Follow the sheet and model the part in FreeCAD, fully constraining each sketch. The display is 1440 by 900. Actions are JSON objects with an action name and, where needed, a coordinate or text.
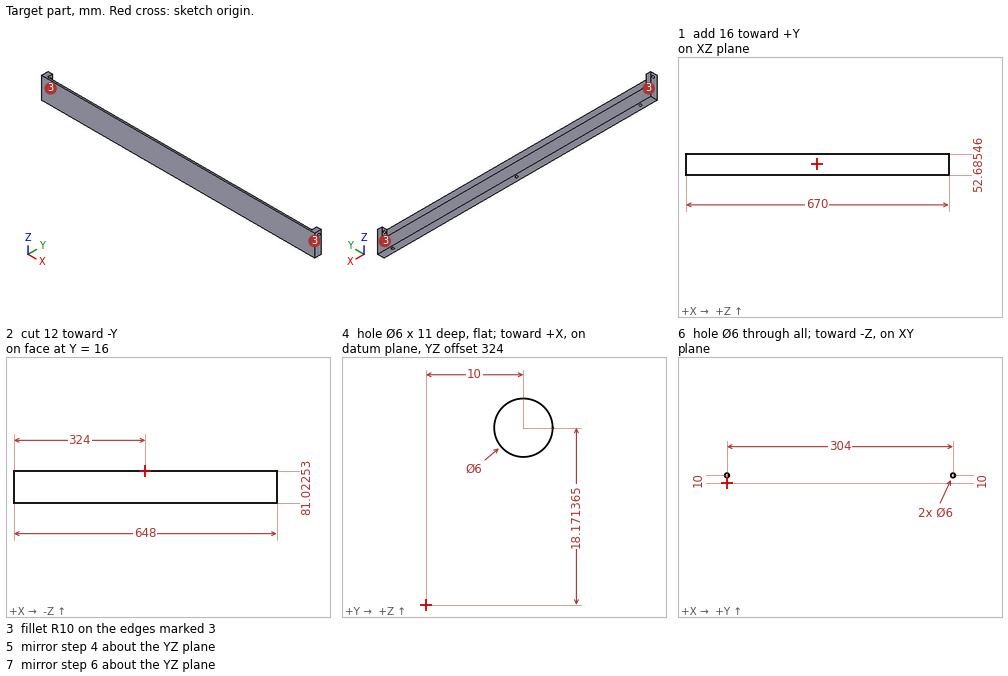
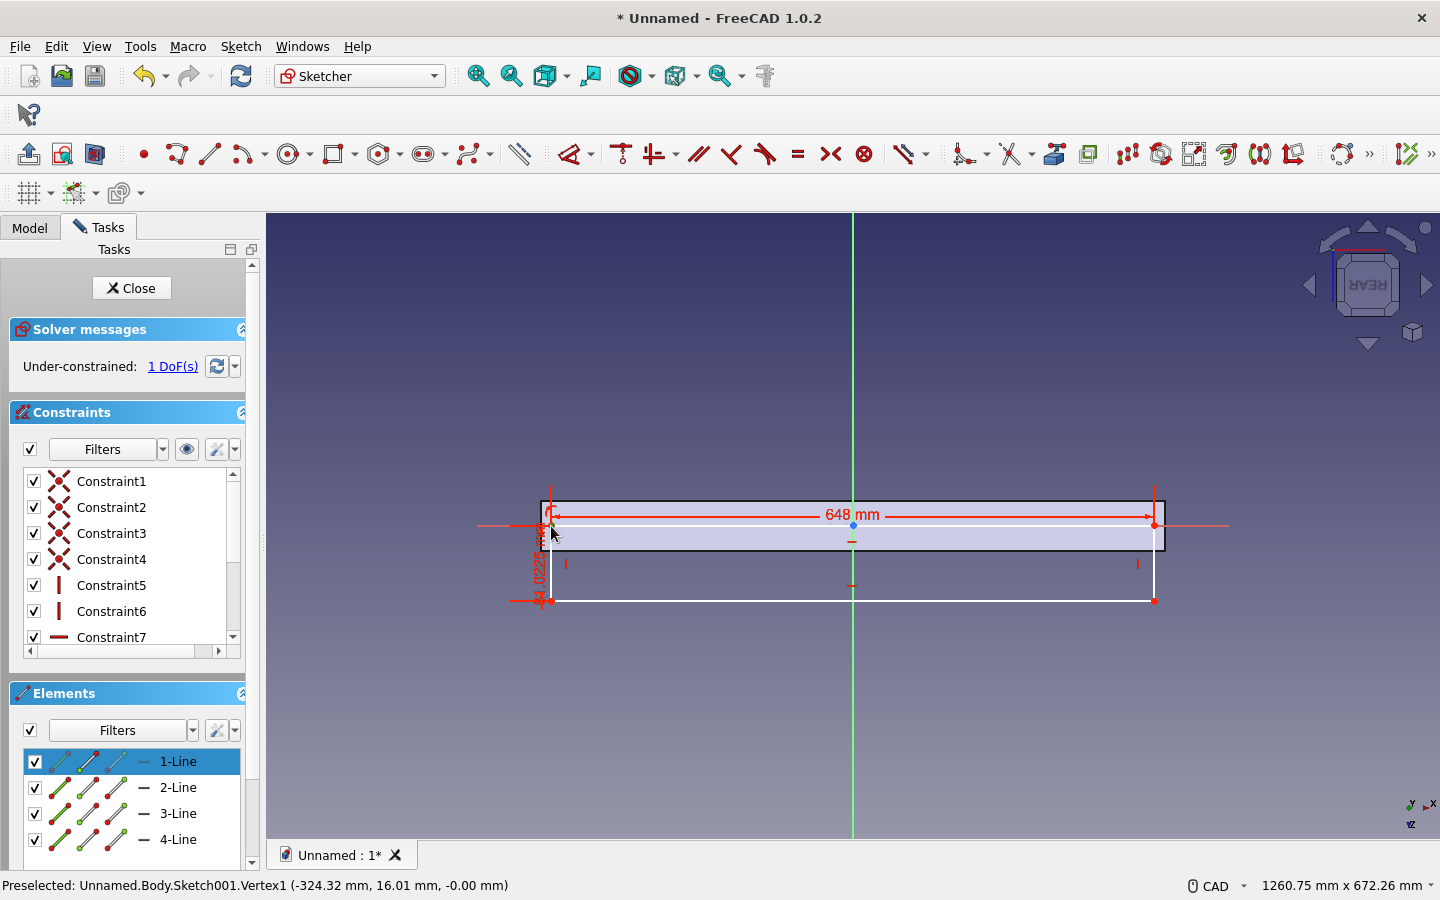
{"action": "key", "text": "l"}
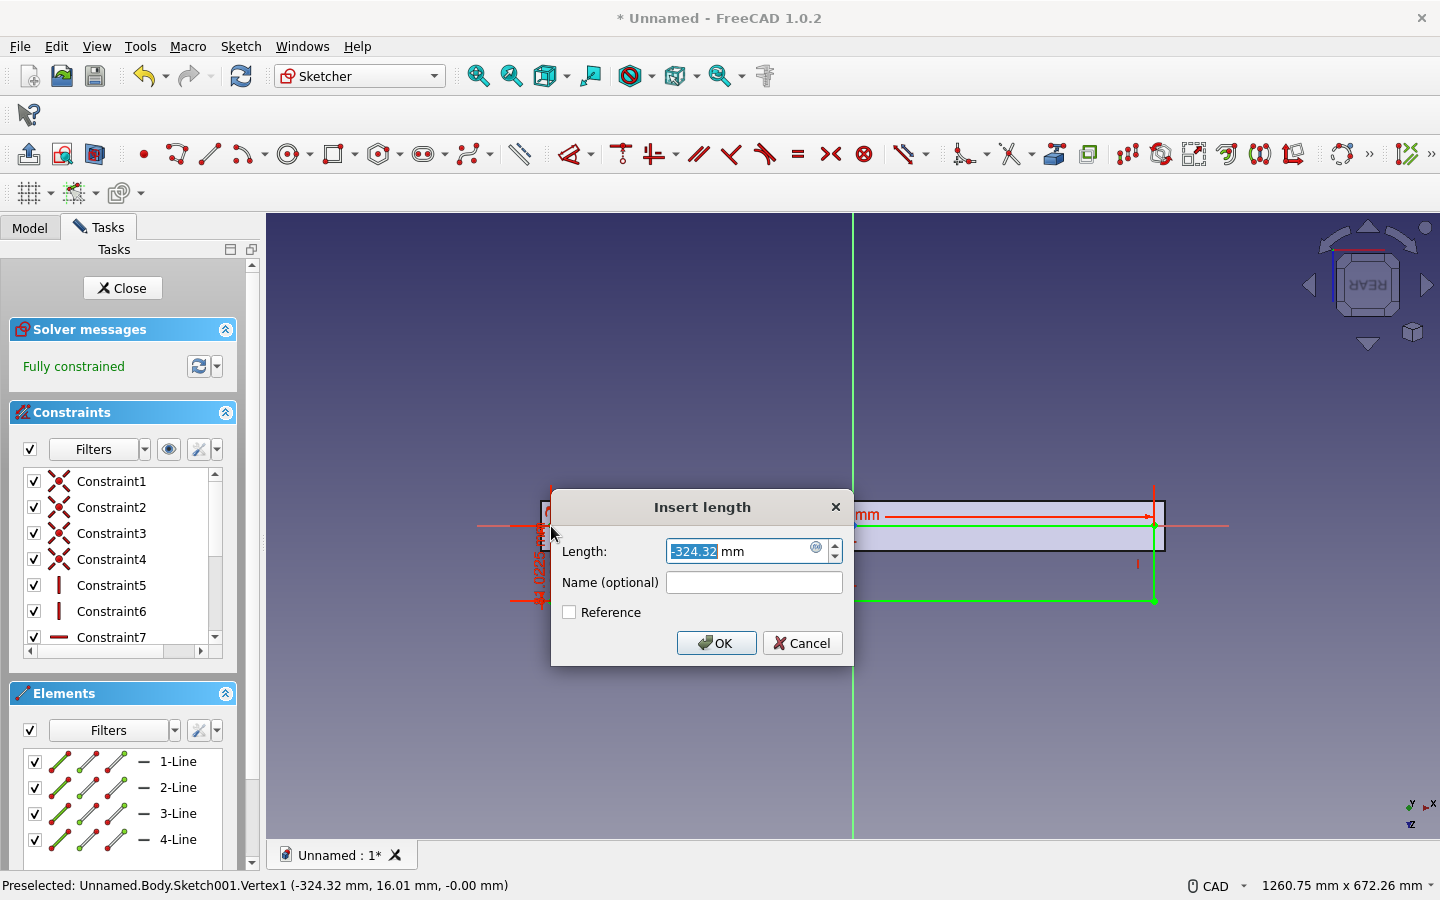
{"action": "type", "text": "-324"}
{"action": "key", "text": "Return"}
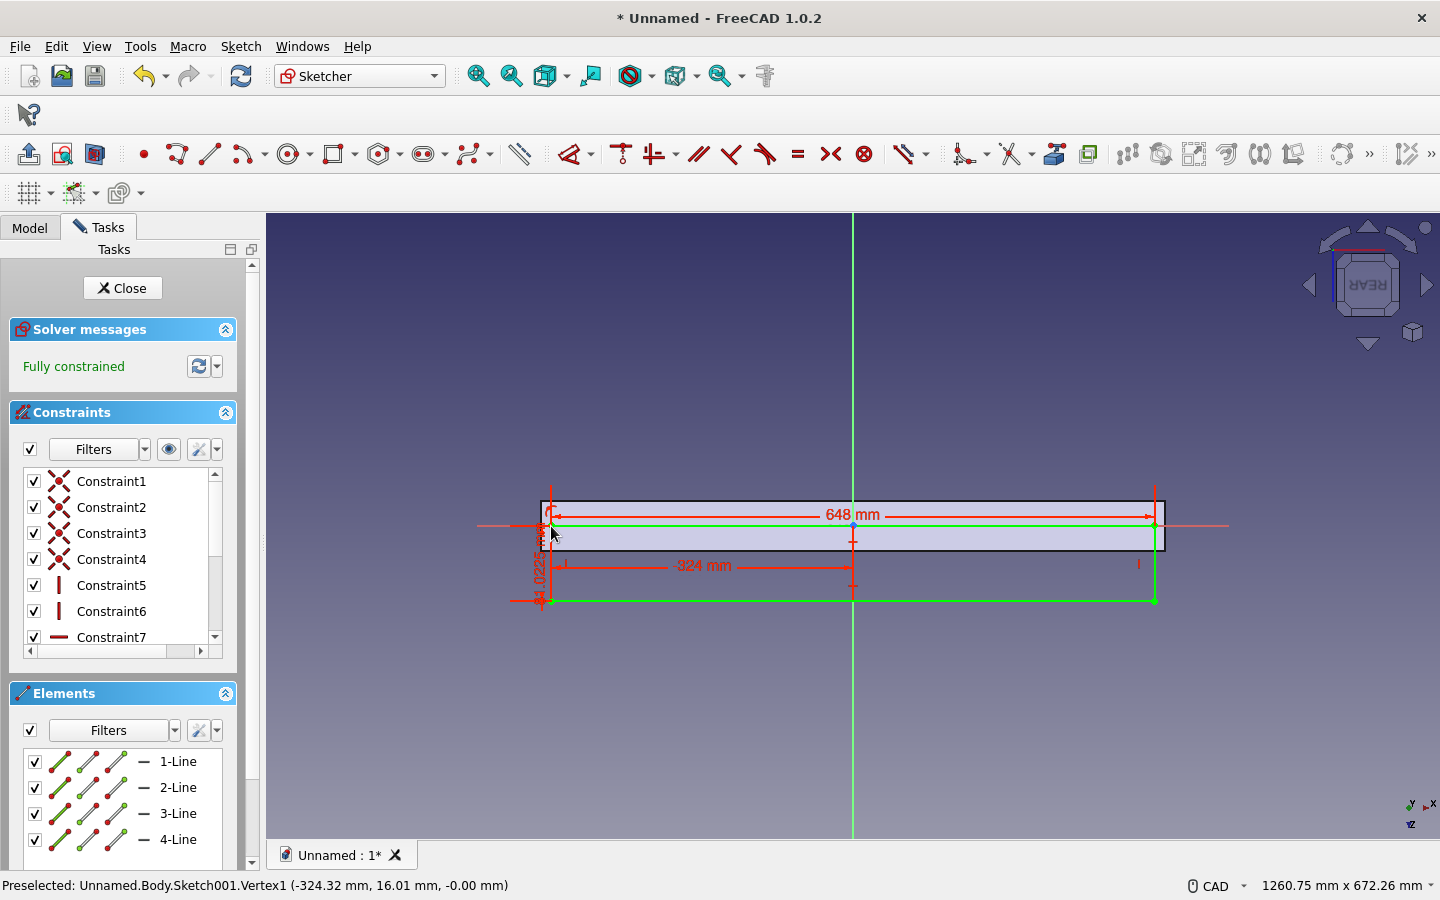
{"action": "left_click", "coordinate": [123, 288]}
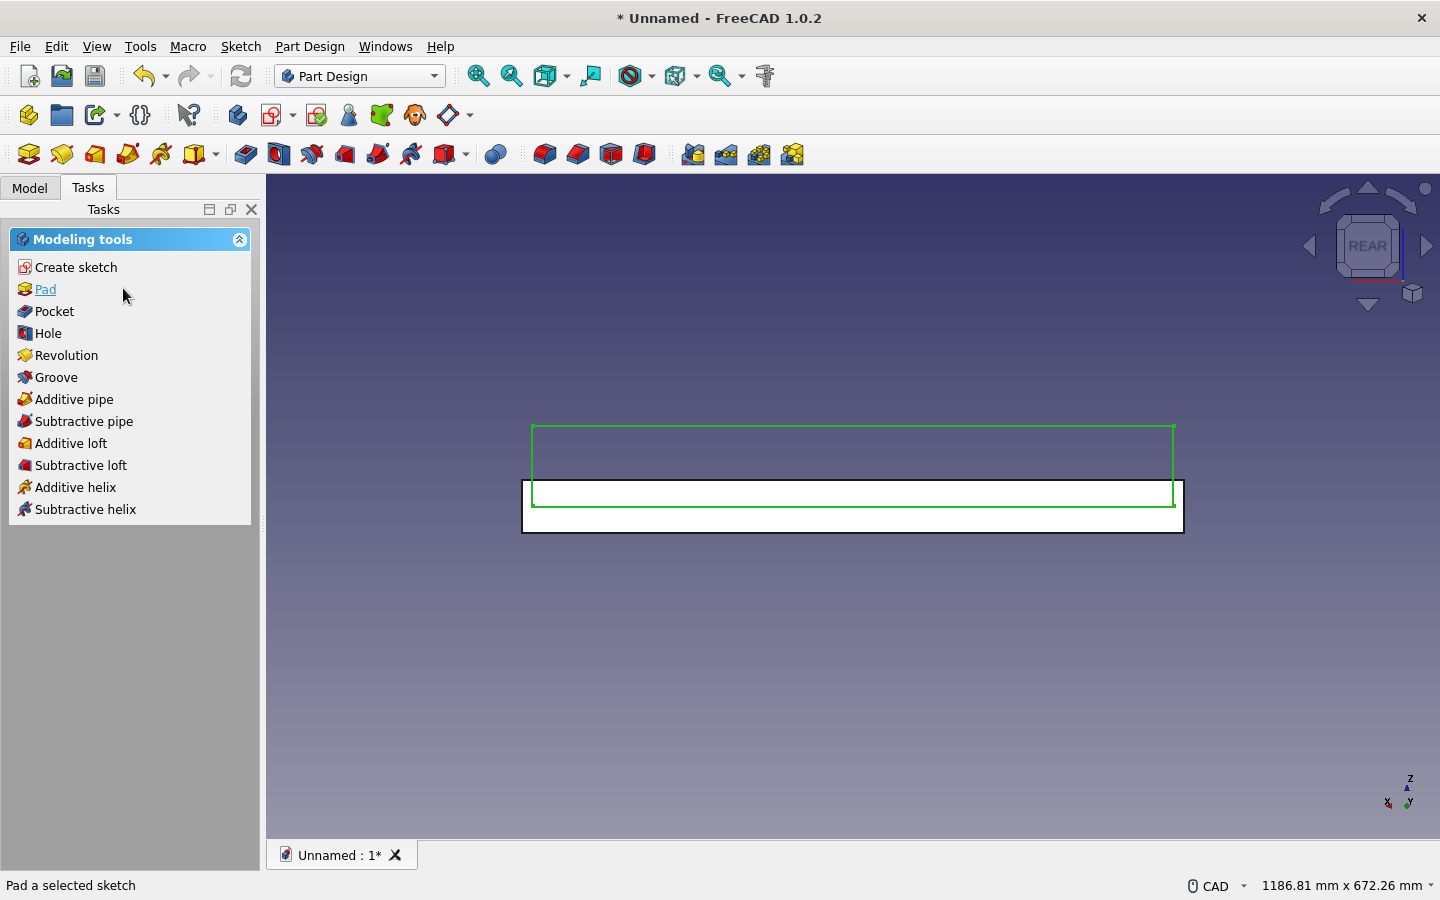
{"action": "left_click", "coordinate": [246, 154]}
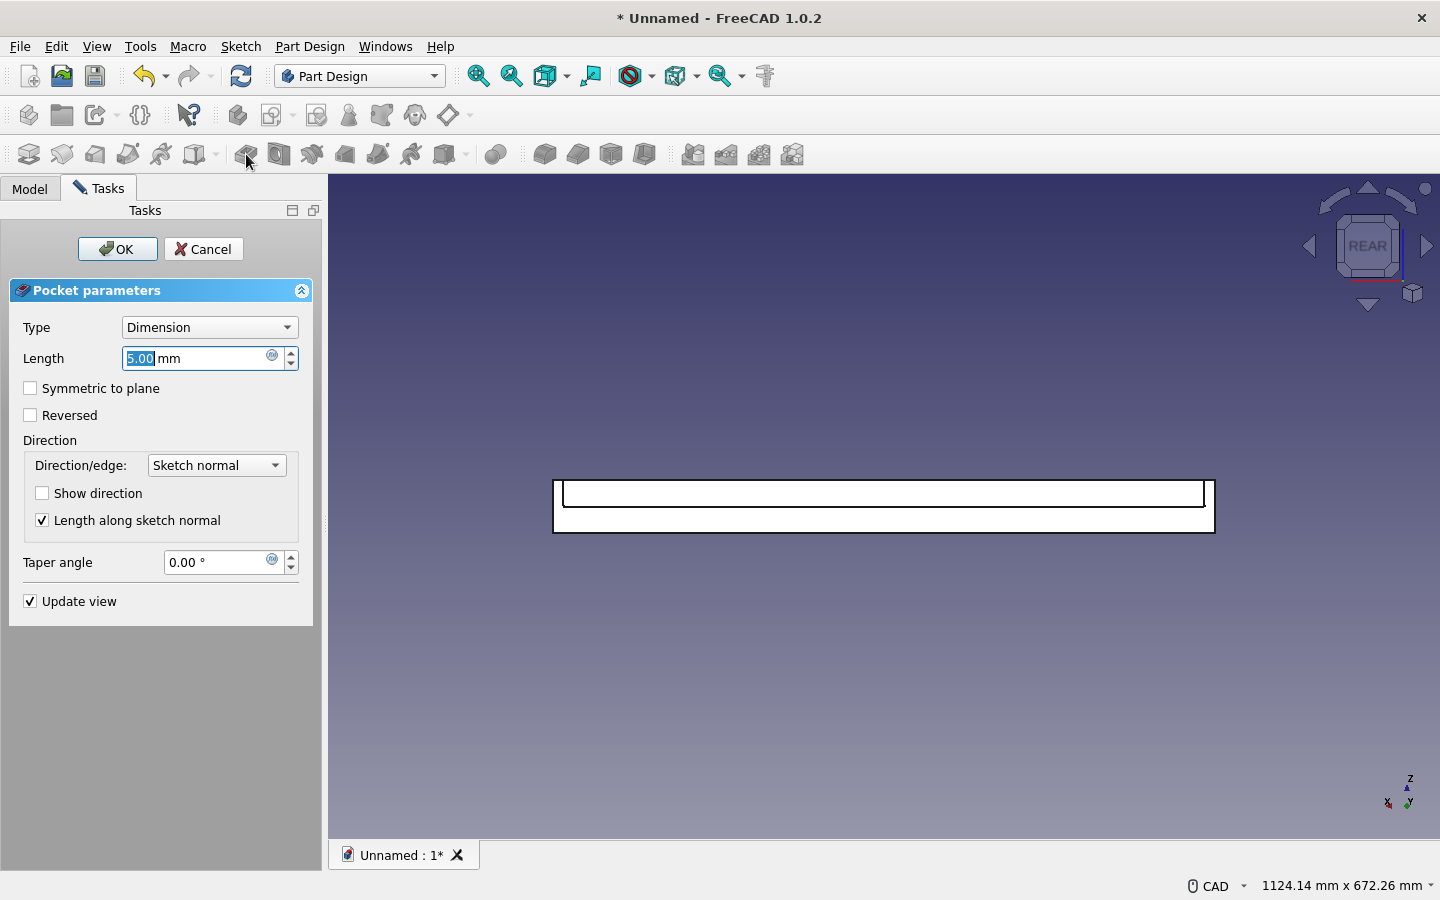
{"action": "type", "text": "12"}
{"action": "key", "text": "Tab"}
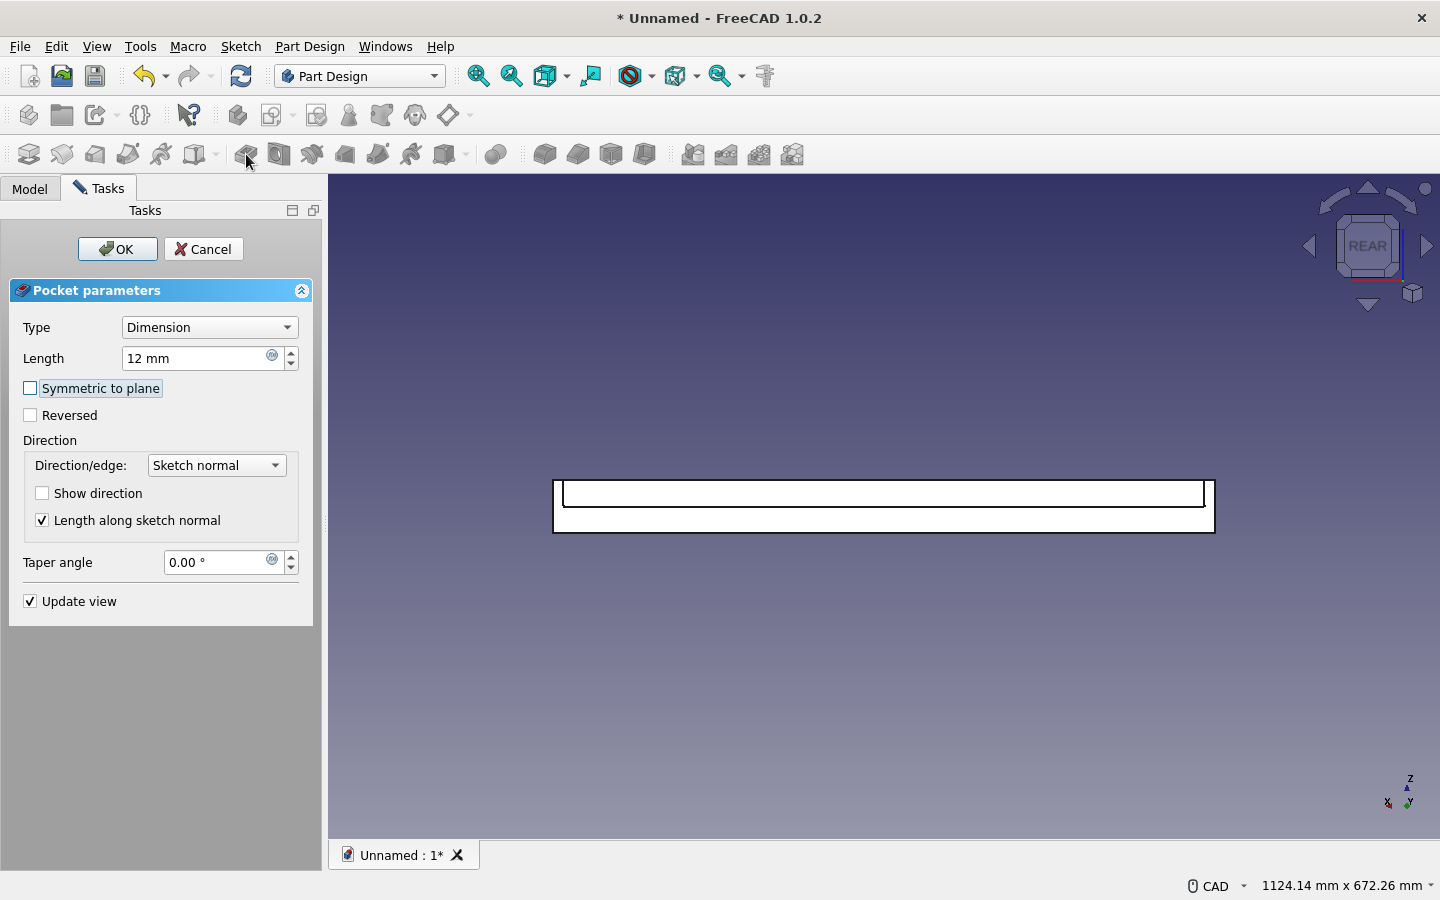
{"action": "left_click", "coordinate": [118, 249]}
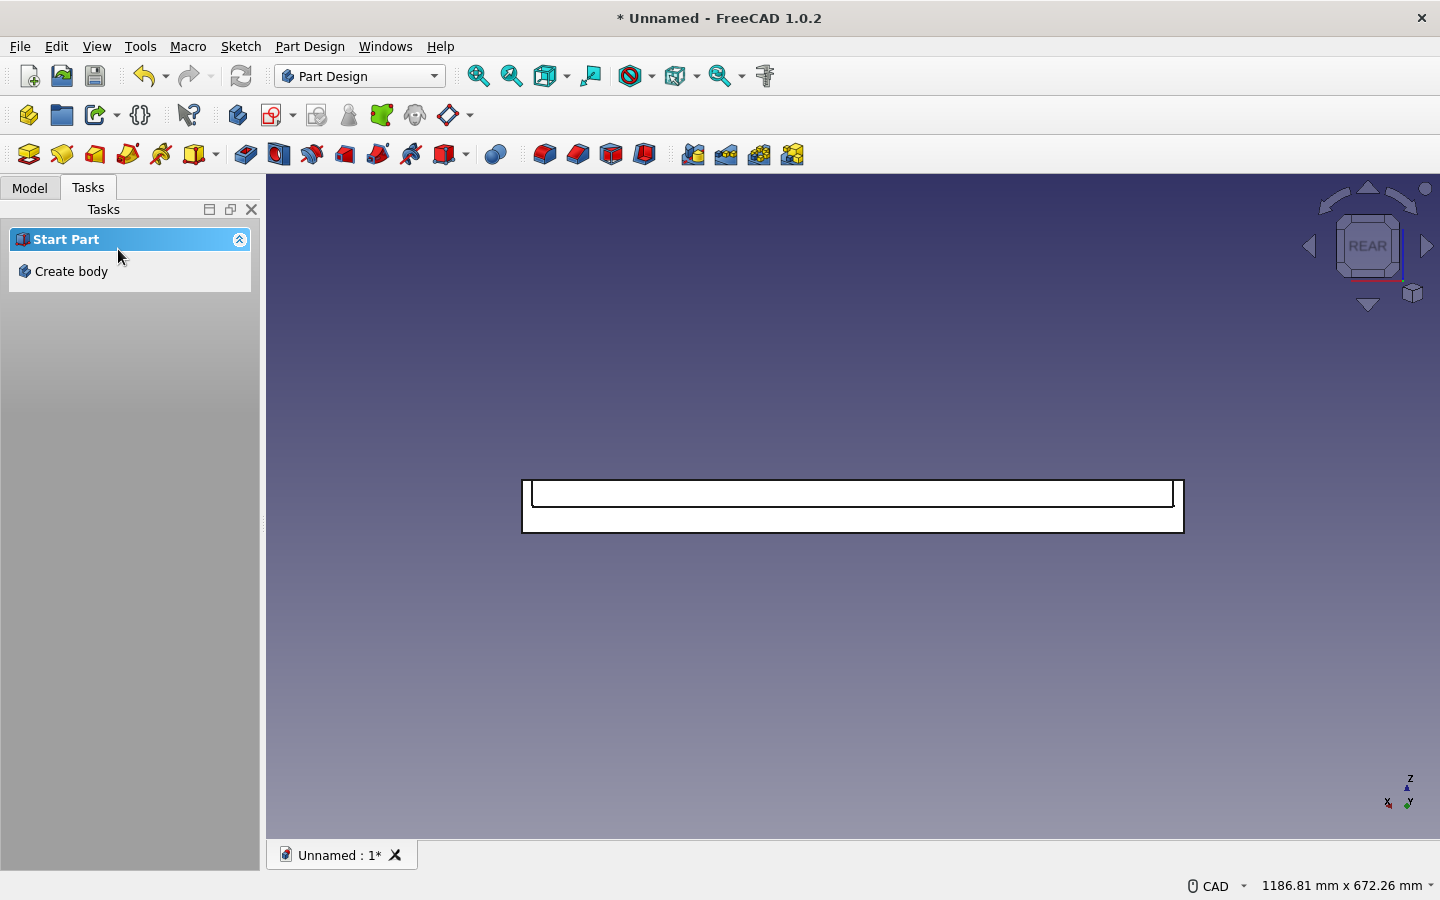
{"action": "scroll", "coordinate": [532, 506], "scroll_direction": "up", "scroll_amount": 7}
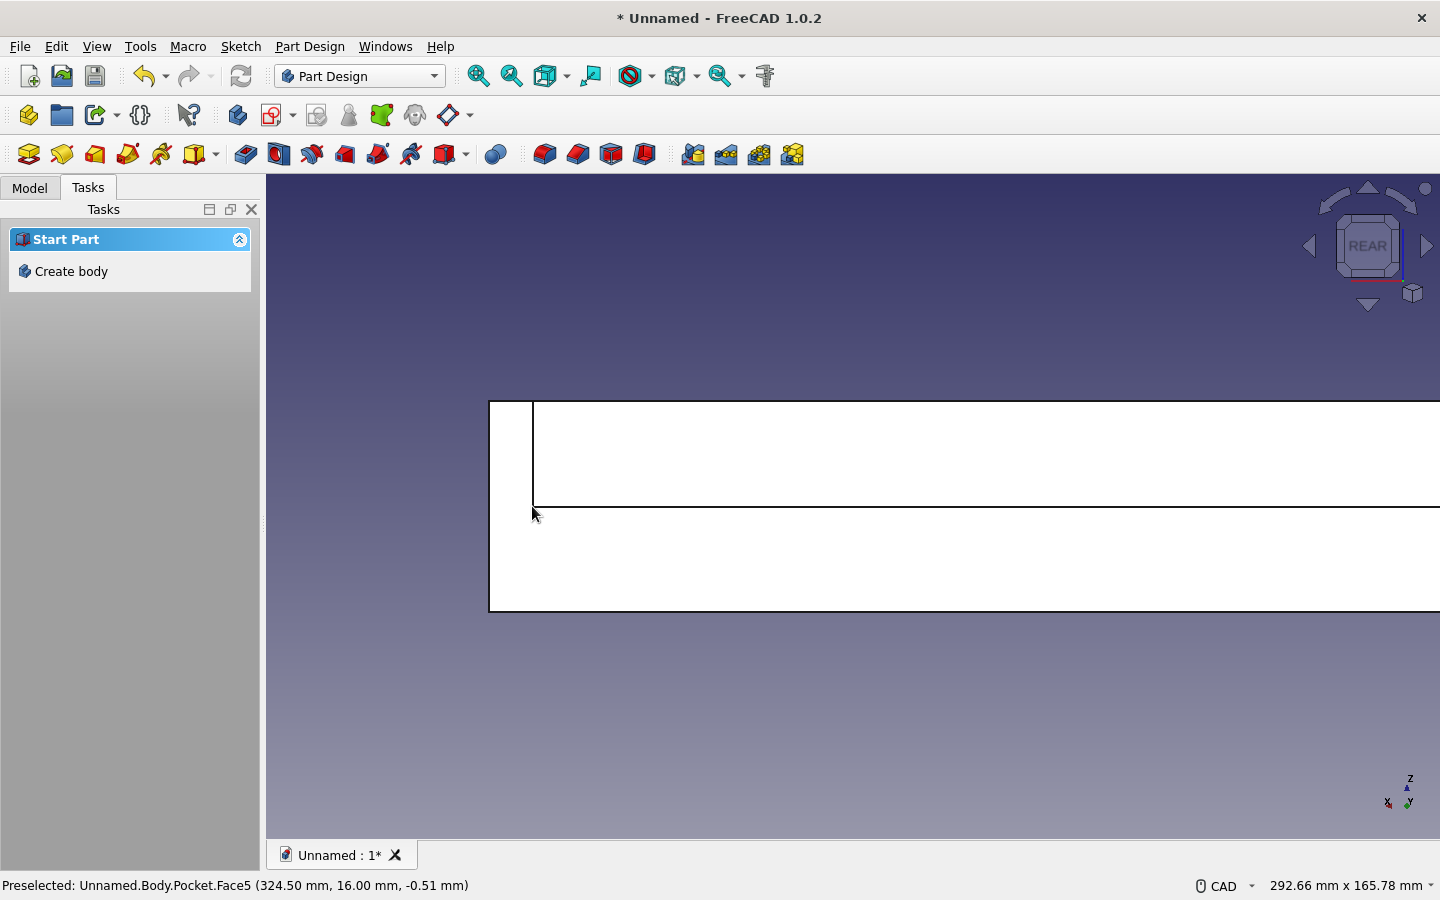
{"action": "key", "text": "v f"}